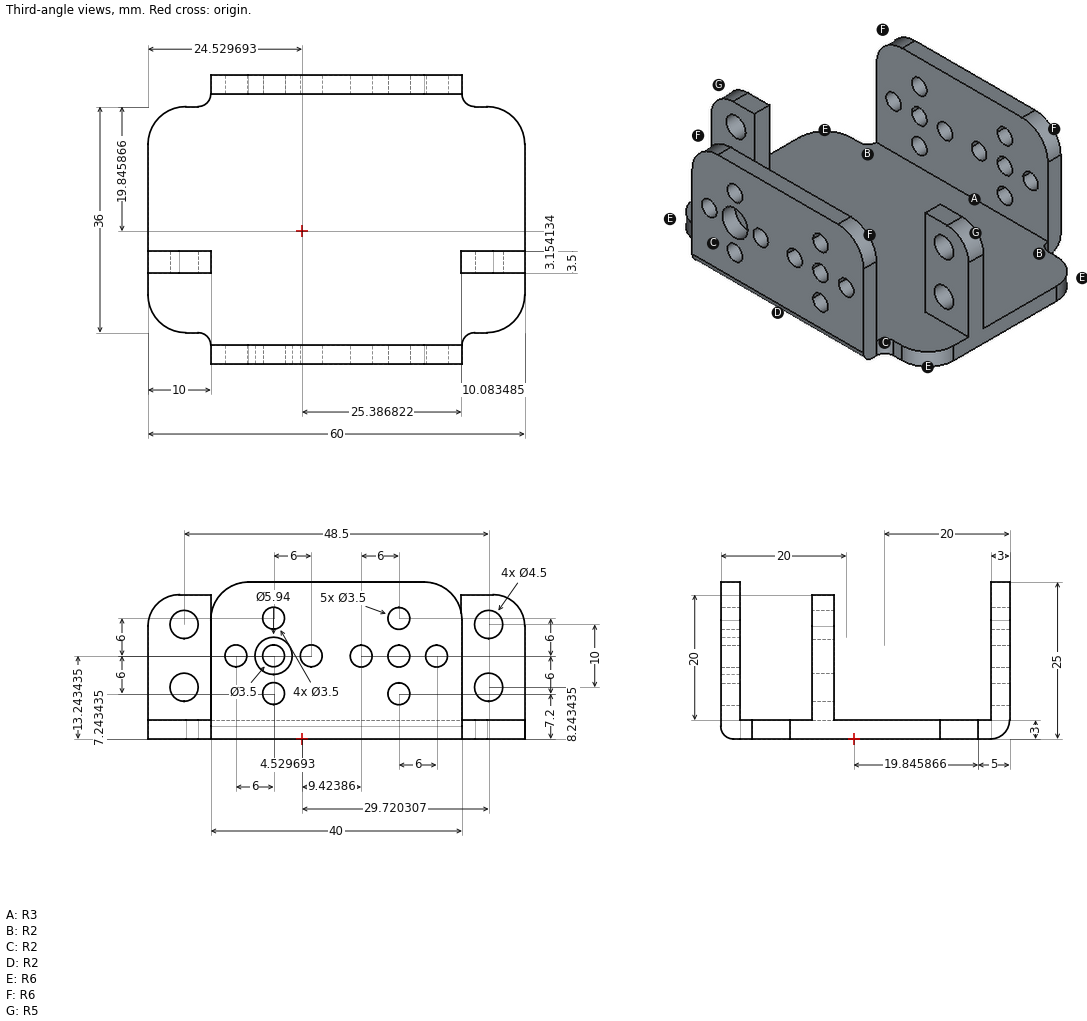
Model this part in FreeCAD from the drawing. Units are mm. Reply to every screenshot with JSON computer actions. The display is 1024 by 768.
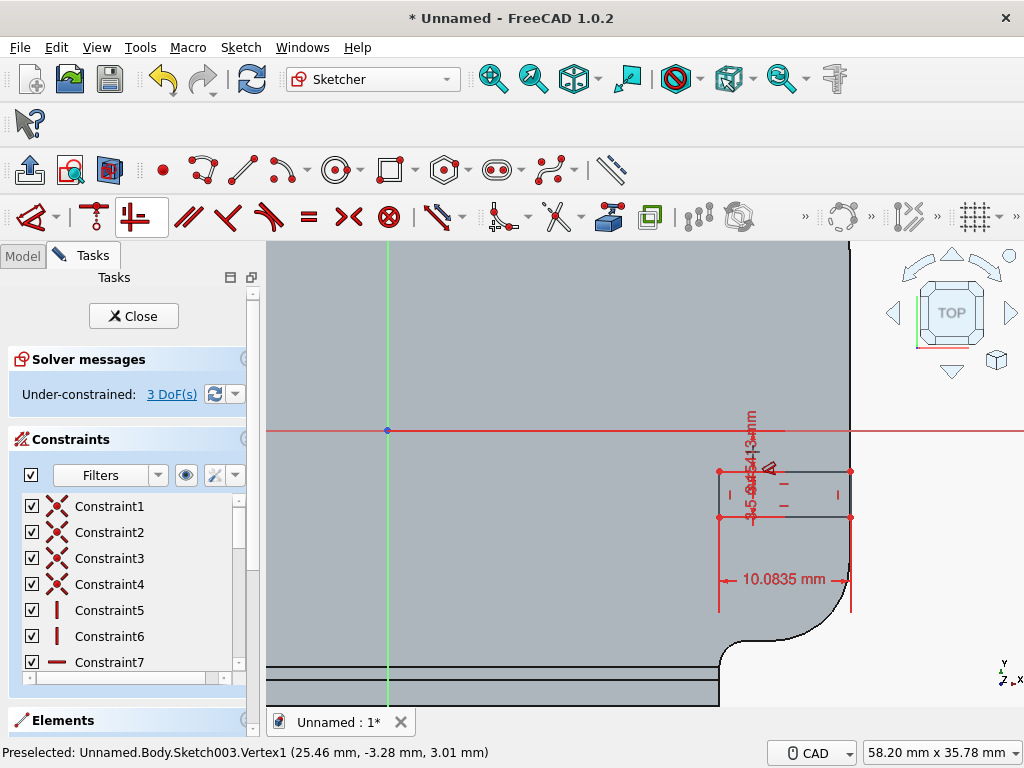
{"action": "scroll", "coordinate": [720, 474], "scroll_direction": "down", "scroll_amount": 3}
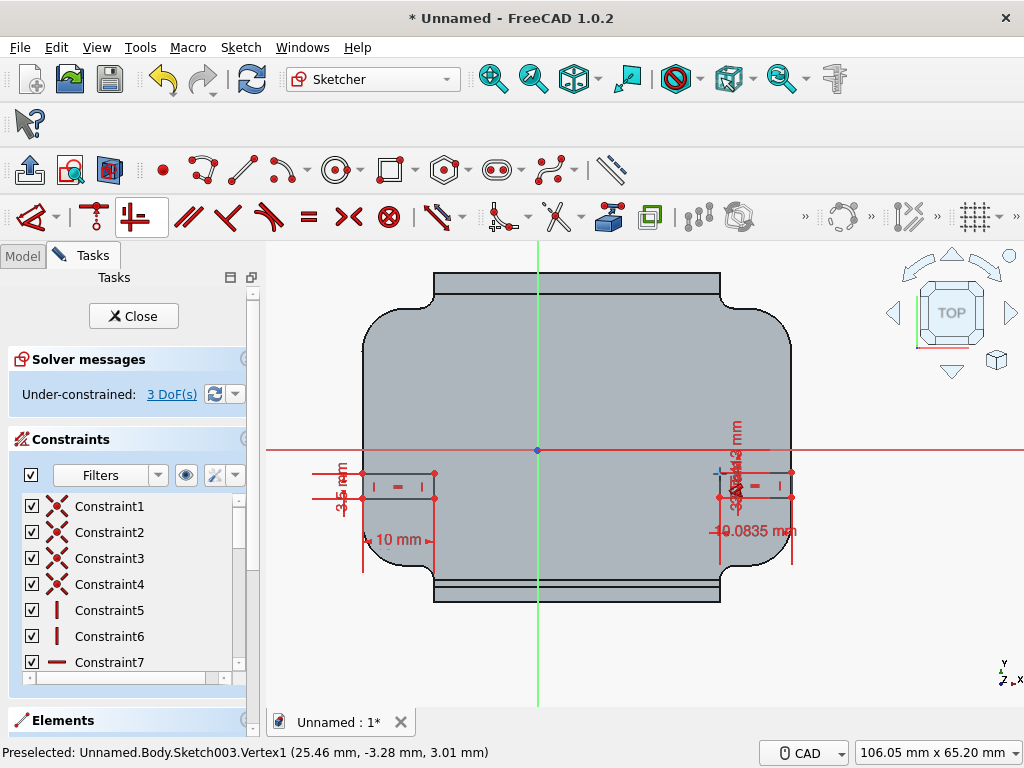
{"action": "scroll", "coordinate": [363, 474], "scroll_direction": "up", "scroll_amount": 3}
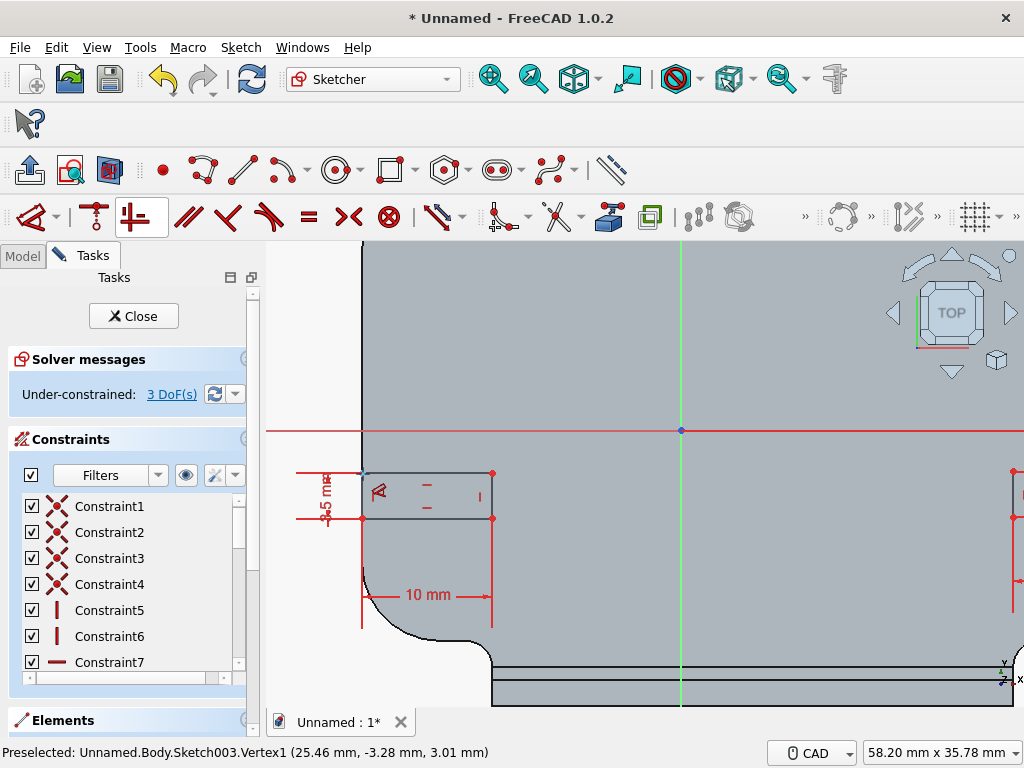
{"action": "left_click", "coordinate": [362, 473]}
{"action": "left_click", "coordinate": [328, 452]}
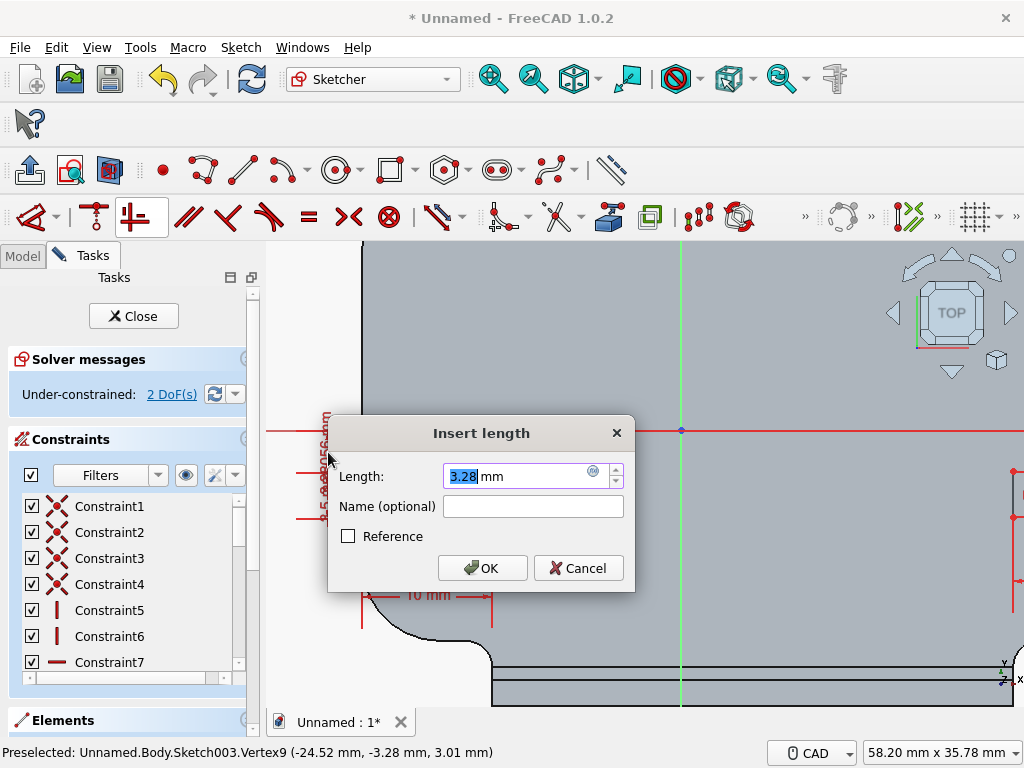
{"action": "type", "text": "3.154134"}
{"action": "key", "text": "Return"}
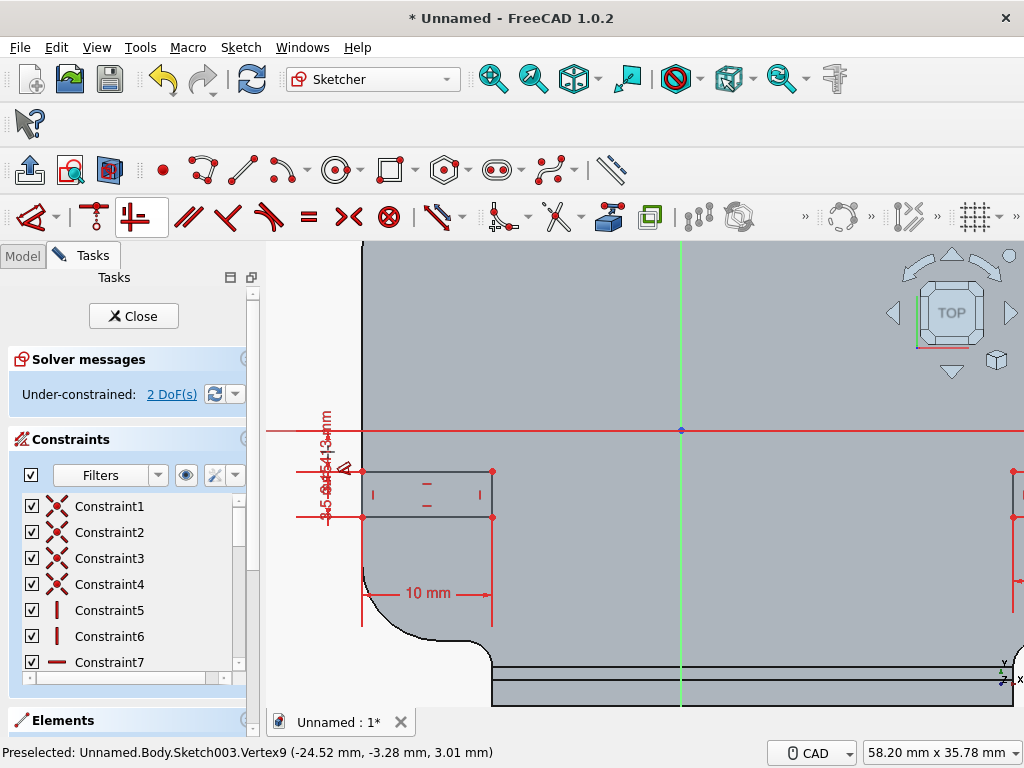
{"action": "scroll", "coordinate": [362, 474], "scroll_direction": "down", "scroll_amount": 3}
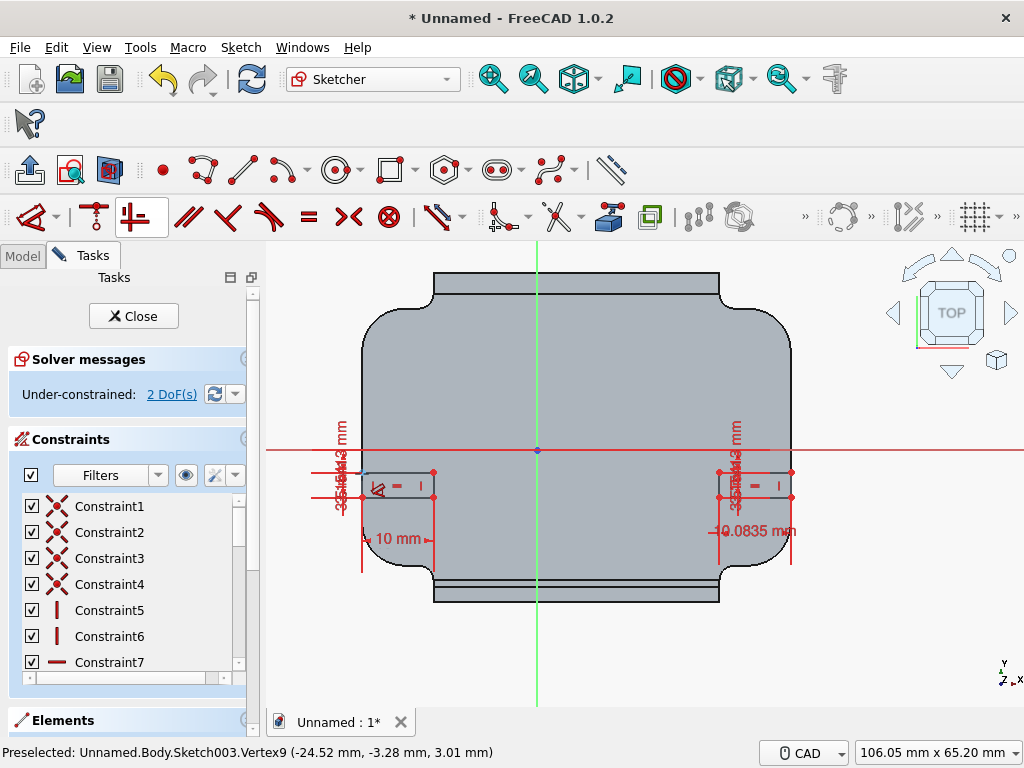
{"action": "left_click", "coordinate": [719, 473]}
{"action": "left_click", "coordinate": [628, 416]}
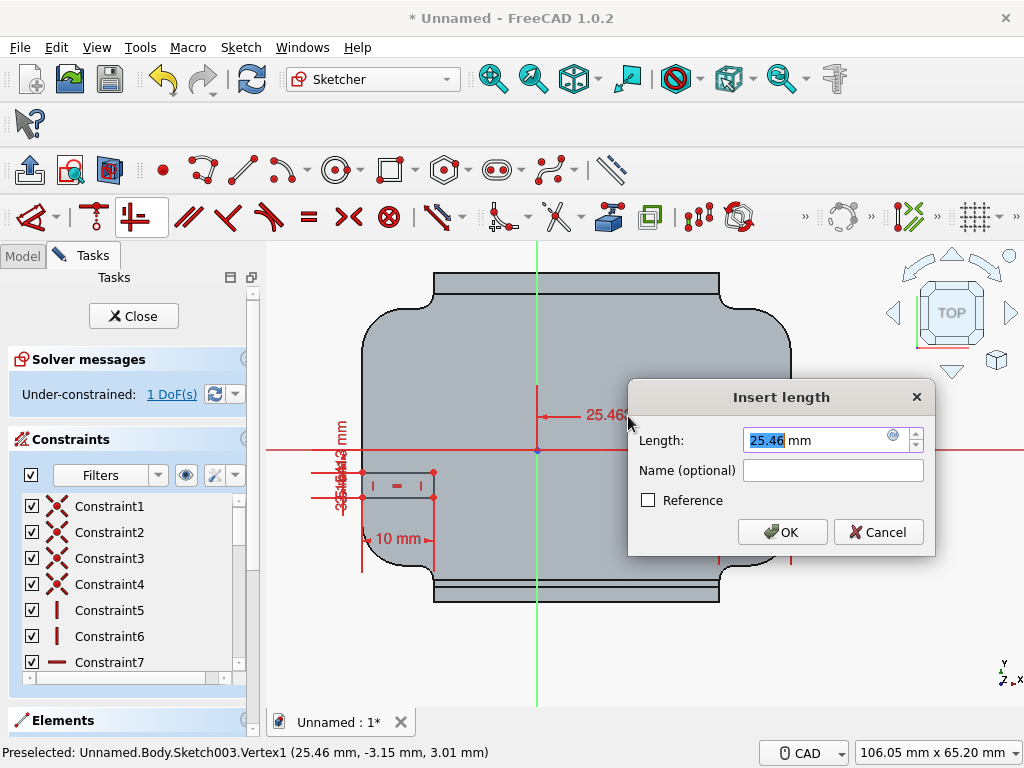
{"action": "type", "text": "25.386822"}
{"action": "key", "text": "Return"}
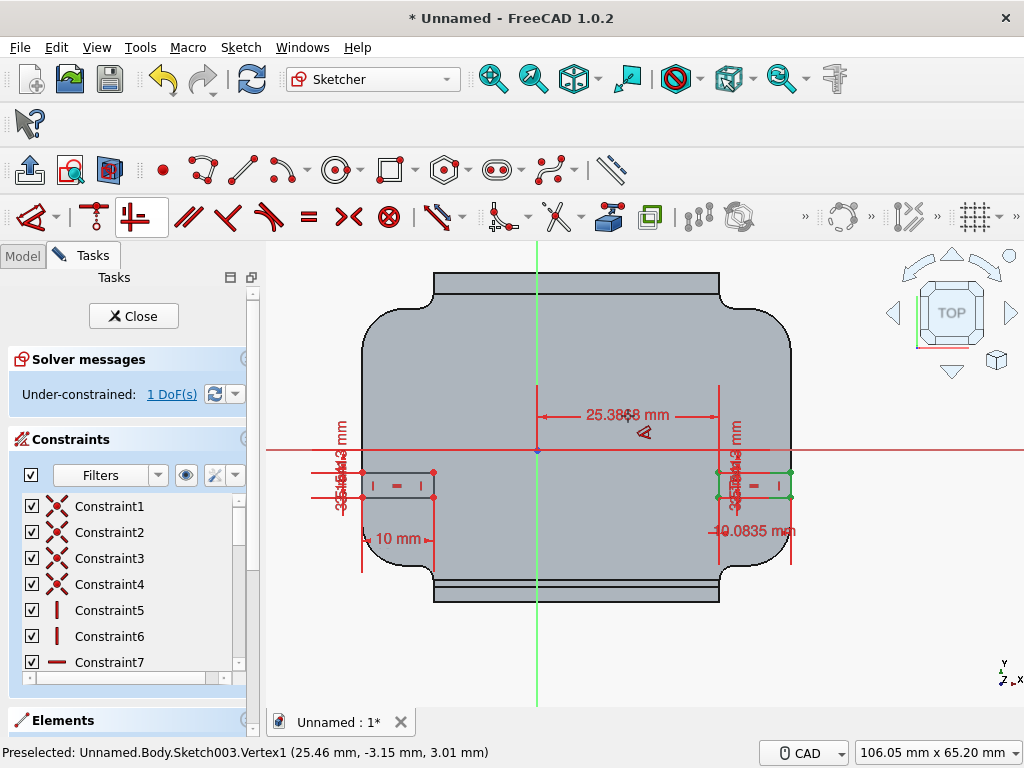
{"action": "left_click", "coordinate": [362, 473]}
{"action": "left_click", "coordinate": [450, 416]}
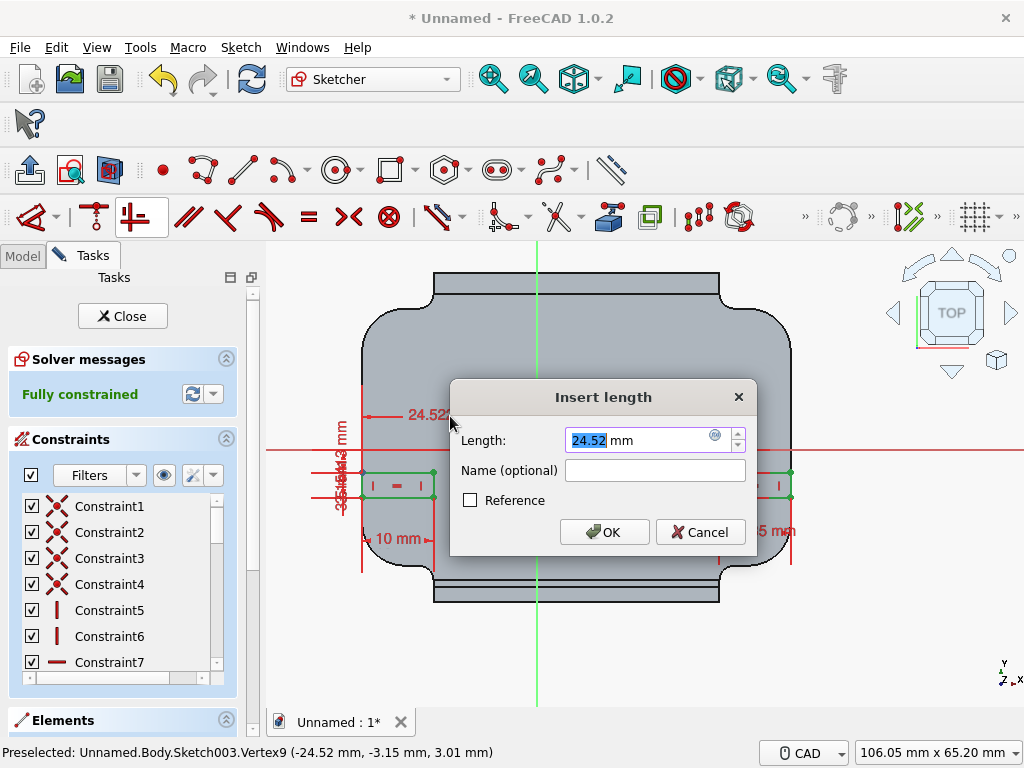
{"action": "type", "text": "24.529693"}
{"action": "key", "text": "Return"}
{"action": "key", "text": "Escape"}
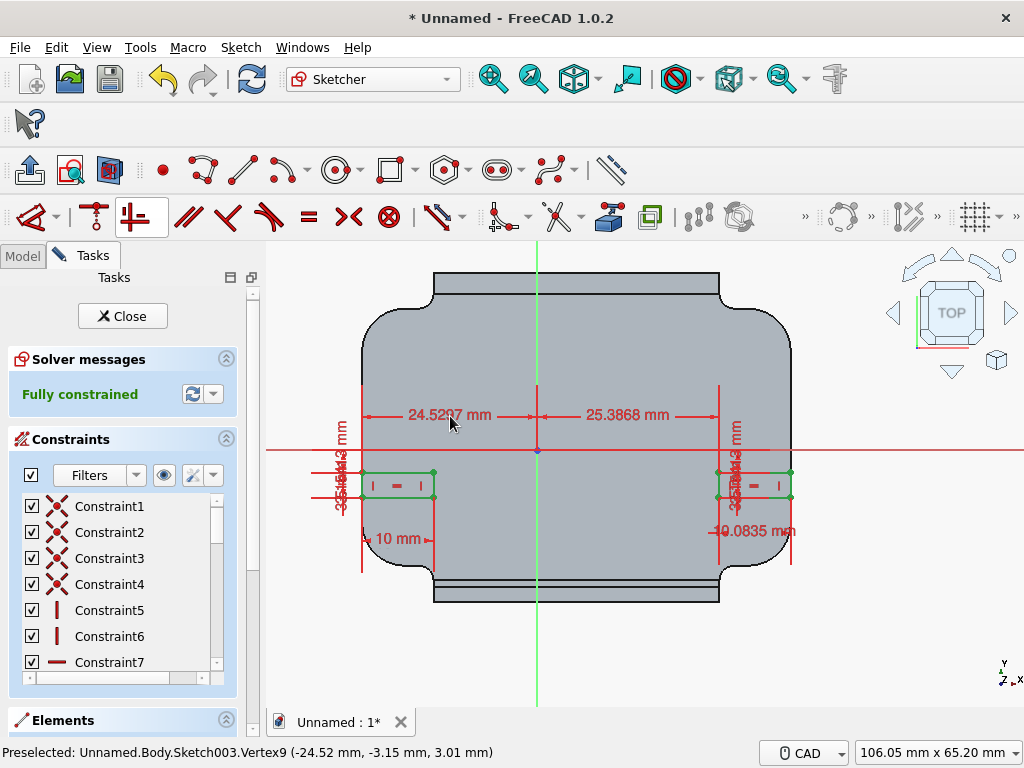
{"action": "left_click", "coordinate": [123, 316]}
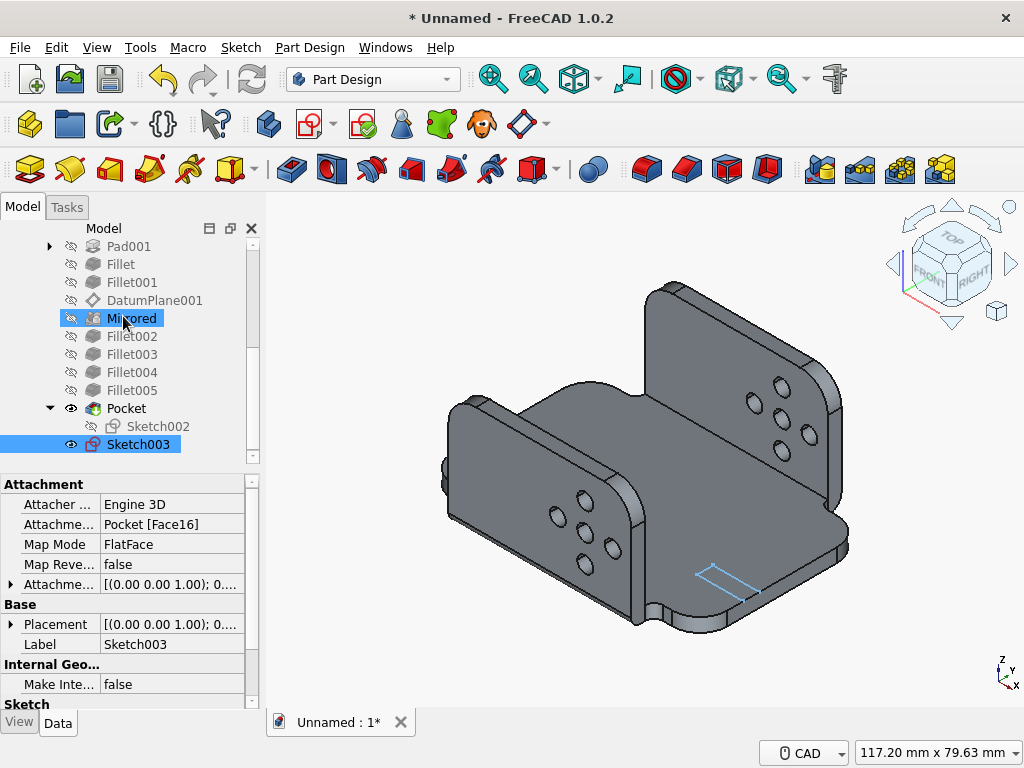
{"action": "left_click", "coordinate": [30, 170]}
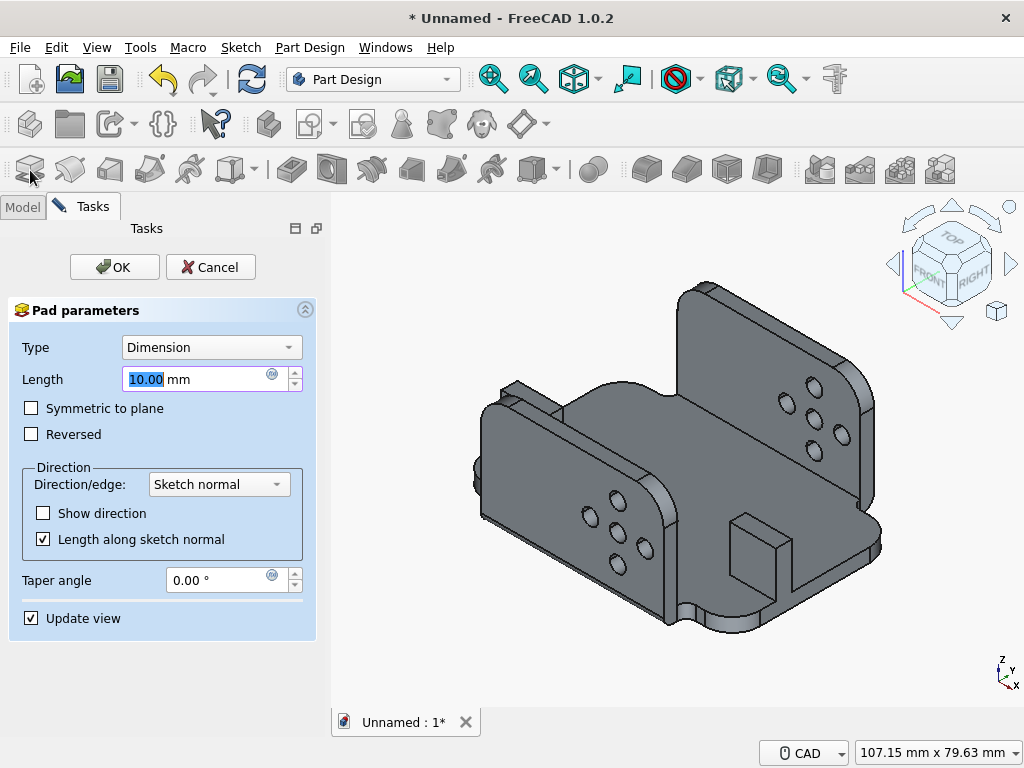
{"action": "type", "text": "20"}
{"action": "key", "text": "Tab"}